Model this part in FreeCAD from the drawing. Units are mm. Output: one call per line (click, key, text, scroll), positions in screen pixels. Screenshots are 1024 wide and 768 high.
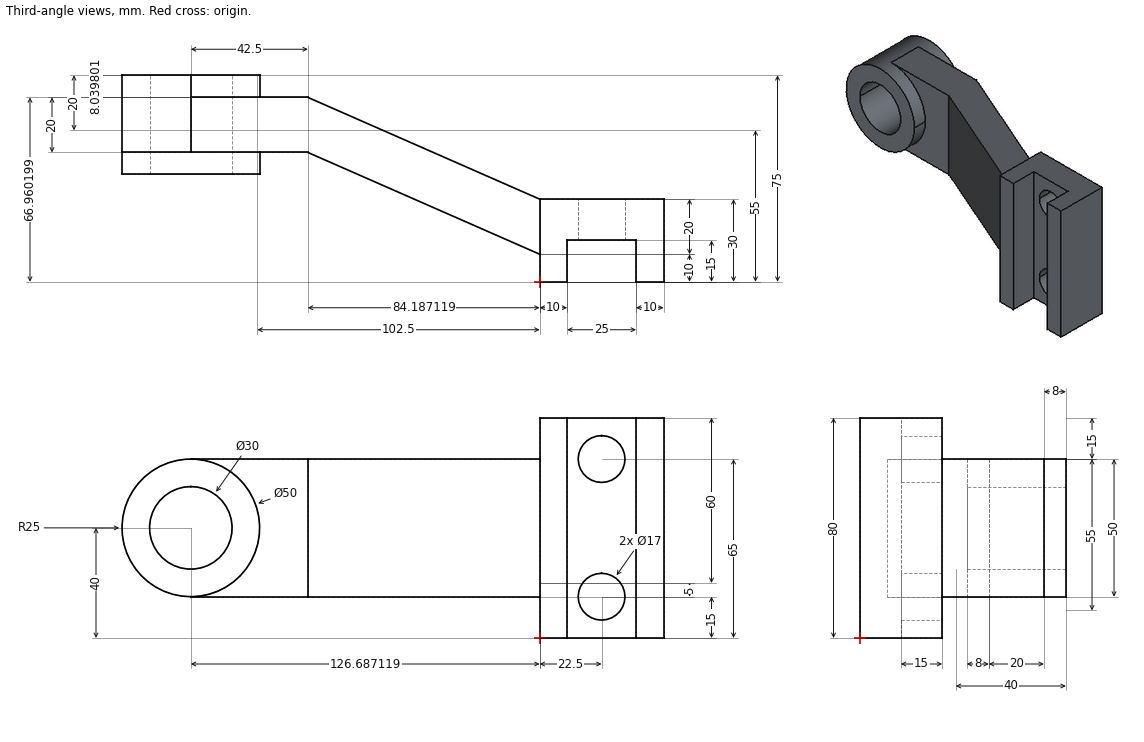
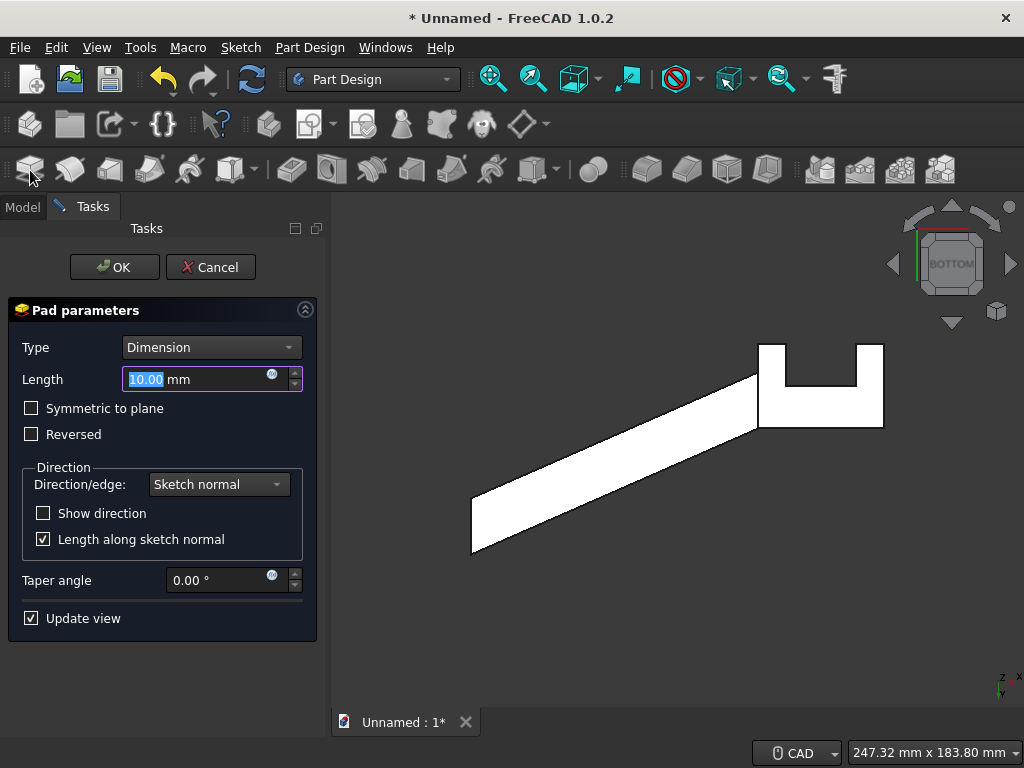
text(5)
key(Tab)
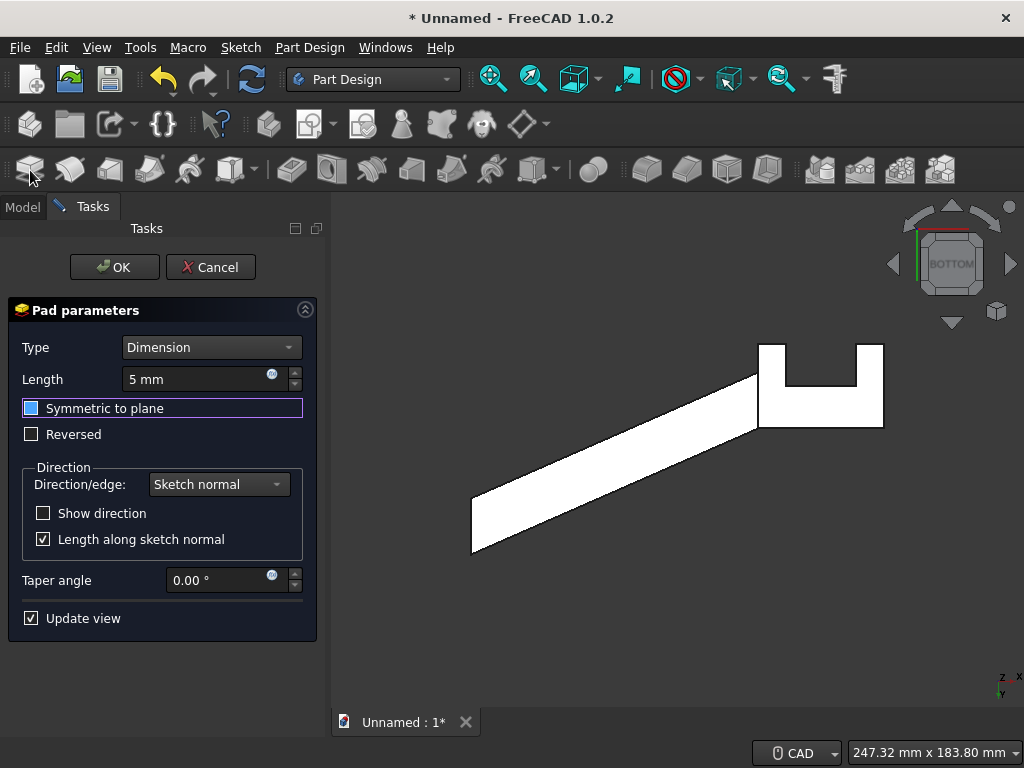
click(115, 267)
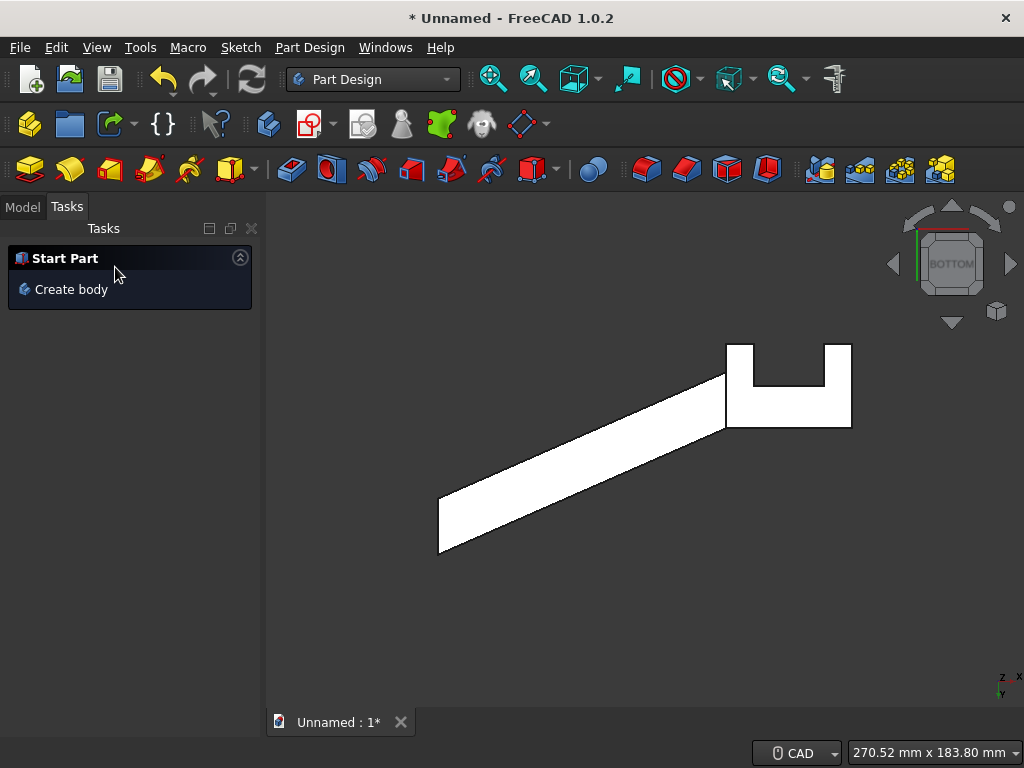
key(4)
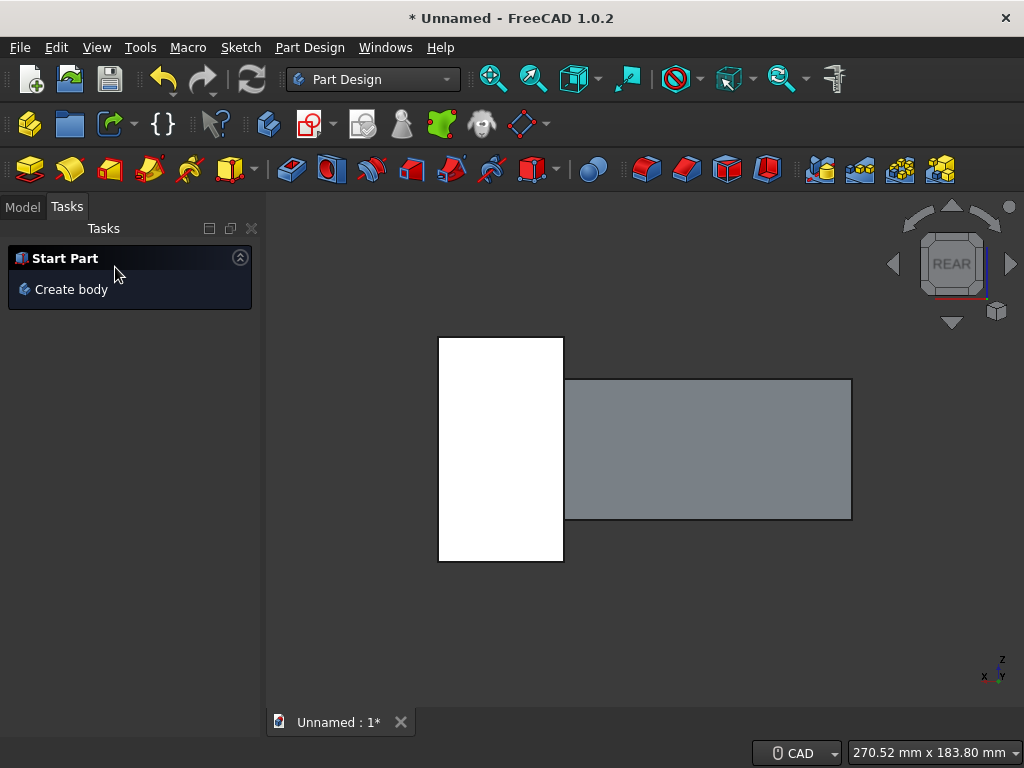
click(501, 416)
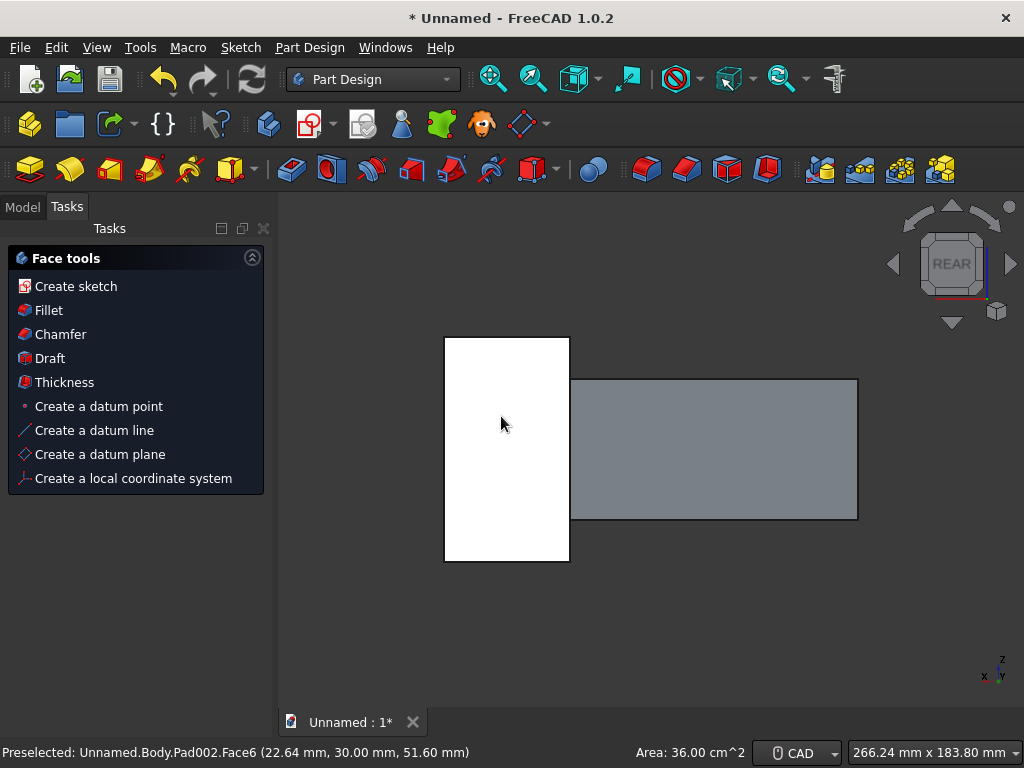
click(310, 124)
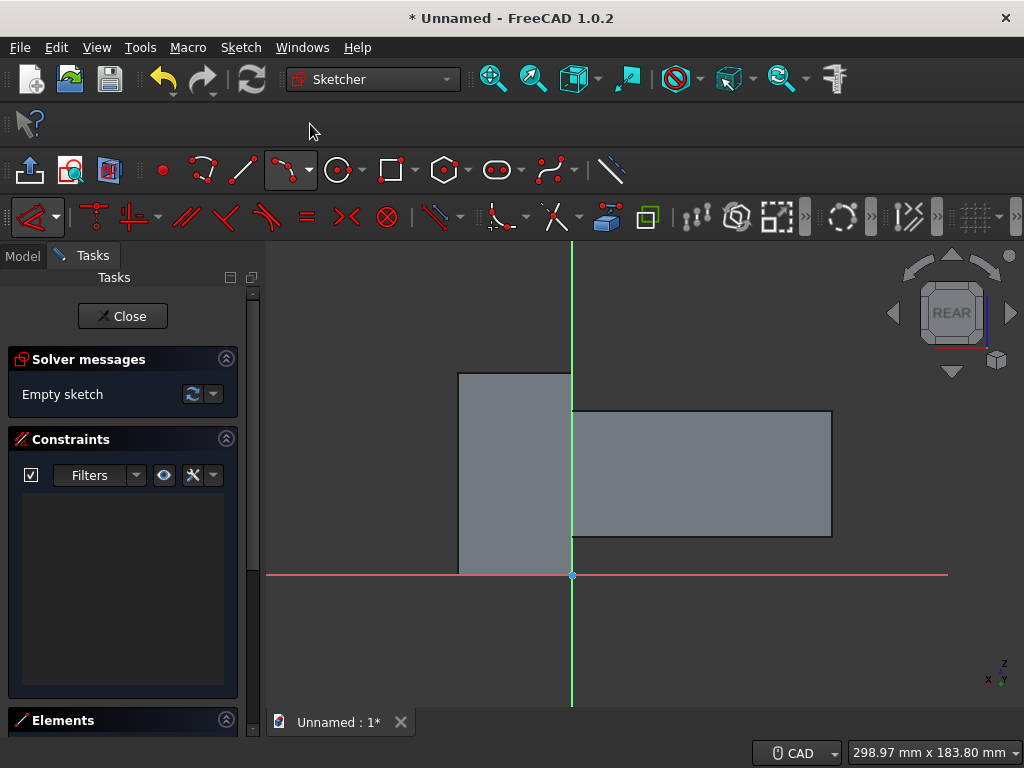
key(q)
key(s)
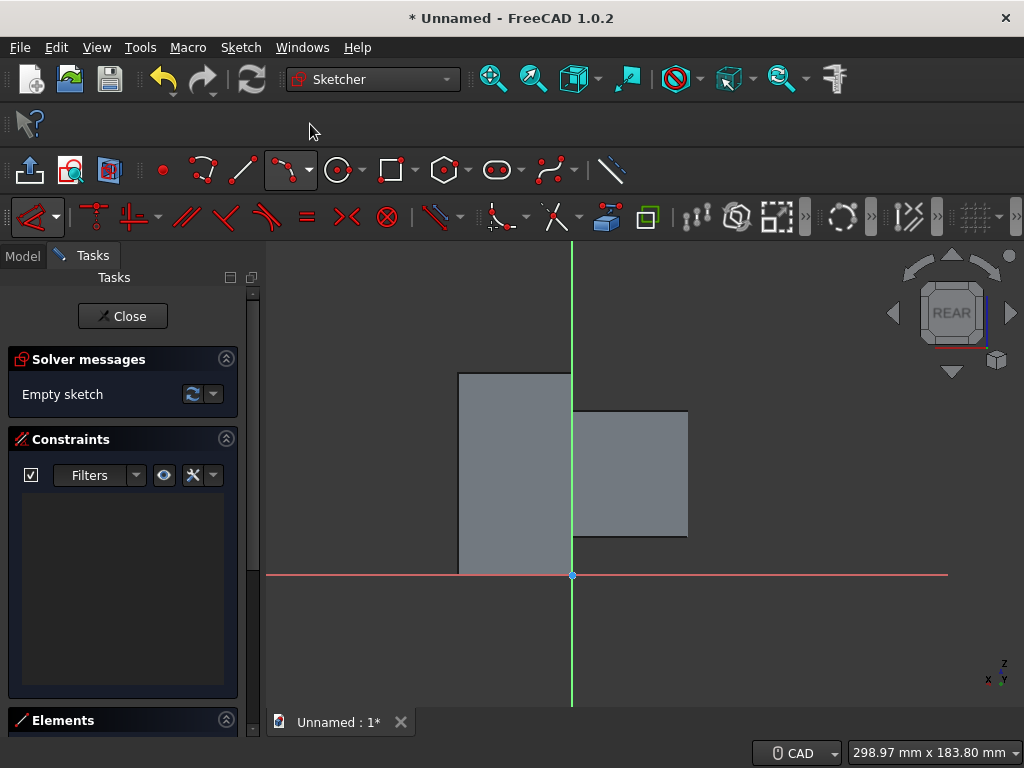
scroll(444, 499, up, 2)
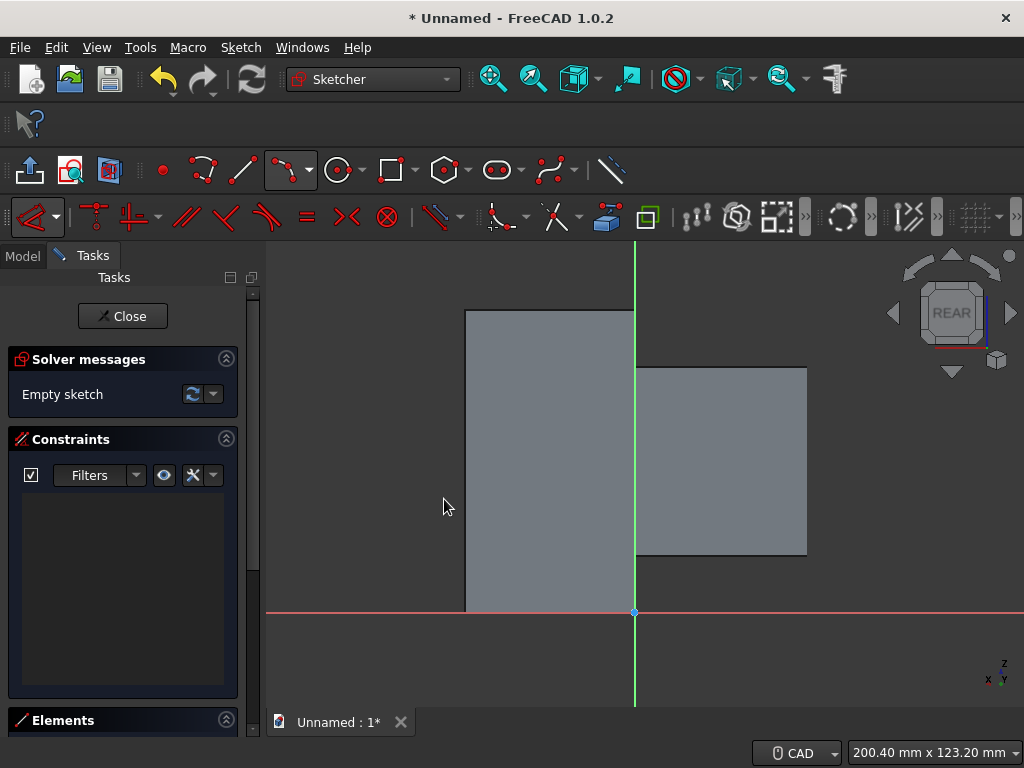
key(g)
key(c)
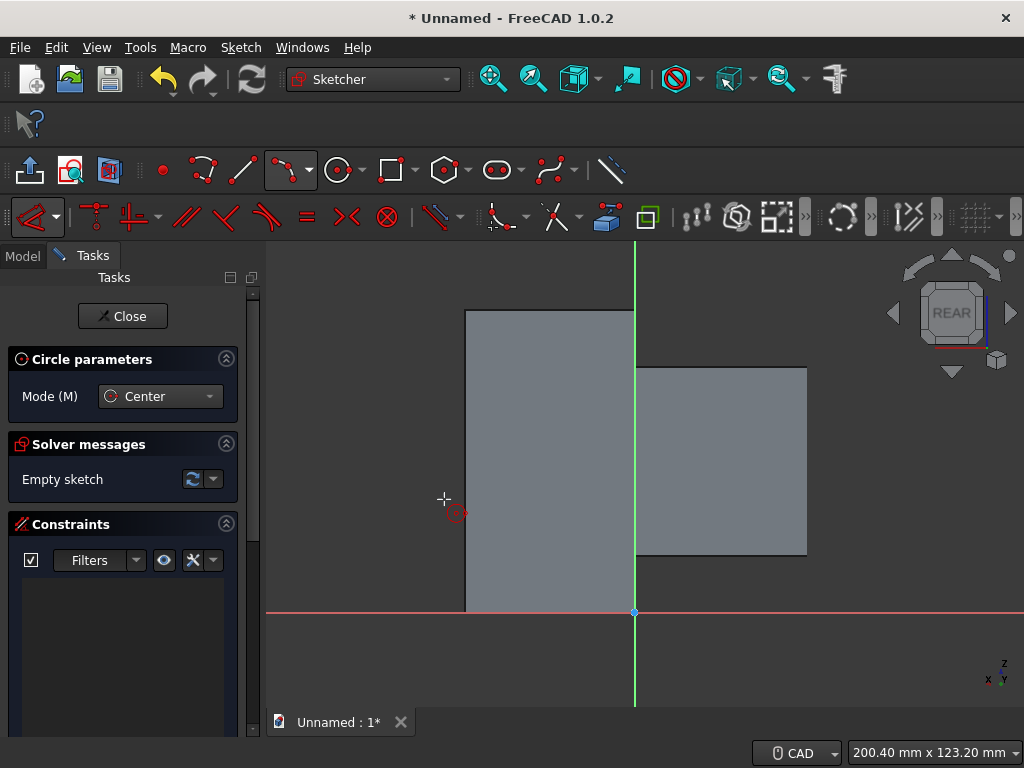
click(550, 556)
move(573, 533)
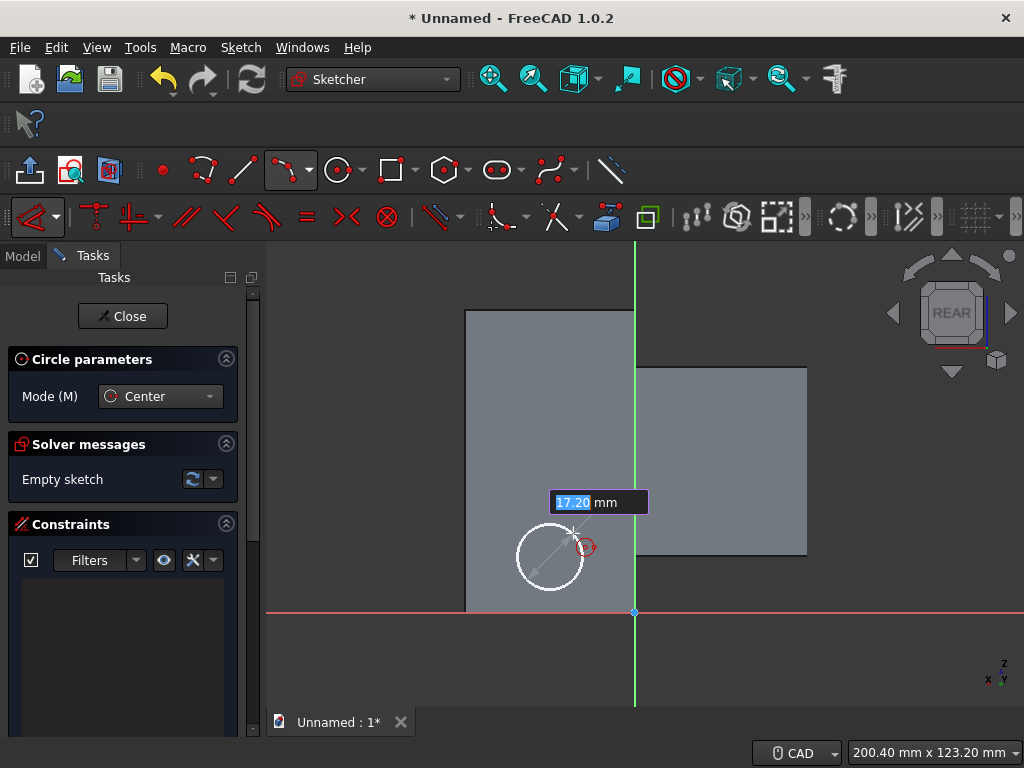
text(17)
key(Return)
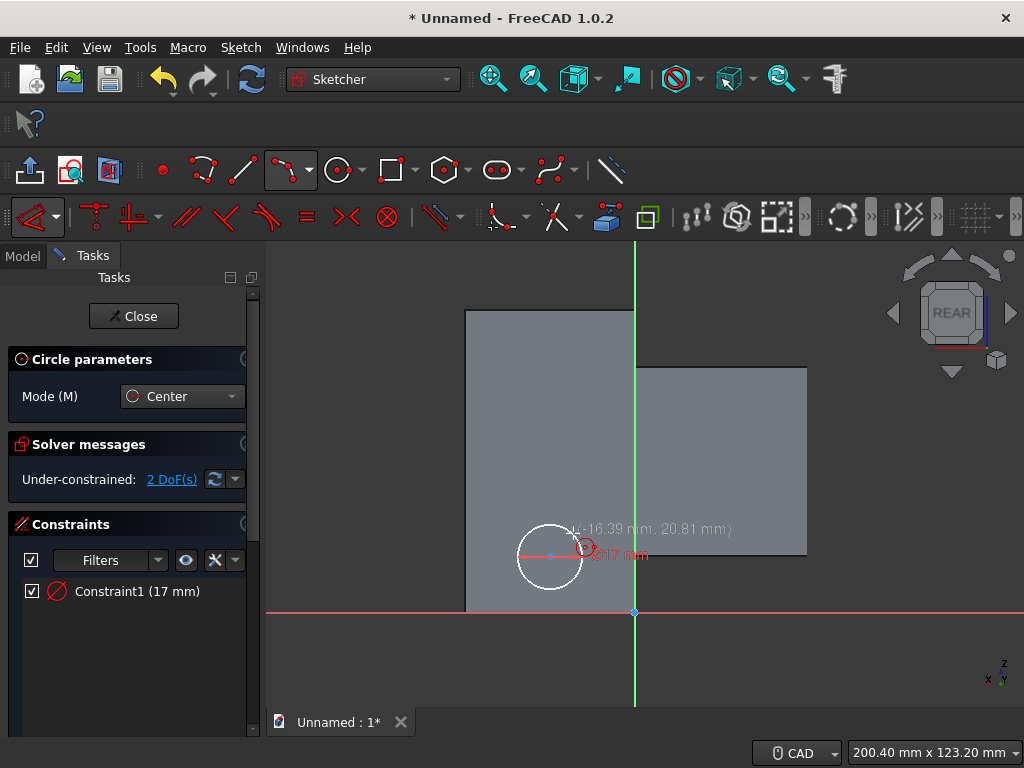
click(550, 367)
move(573, 344)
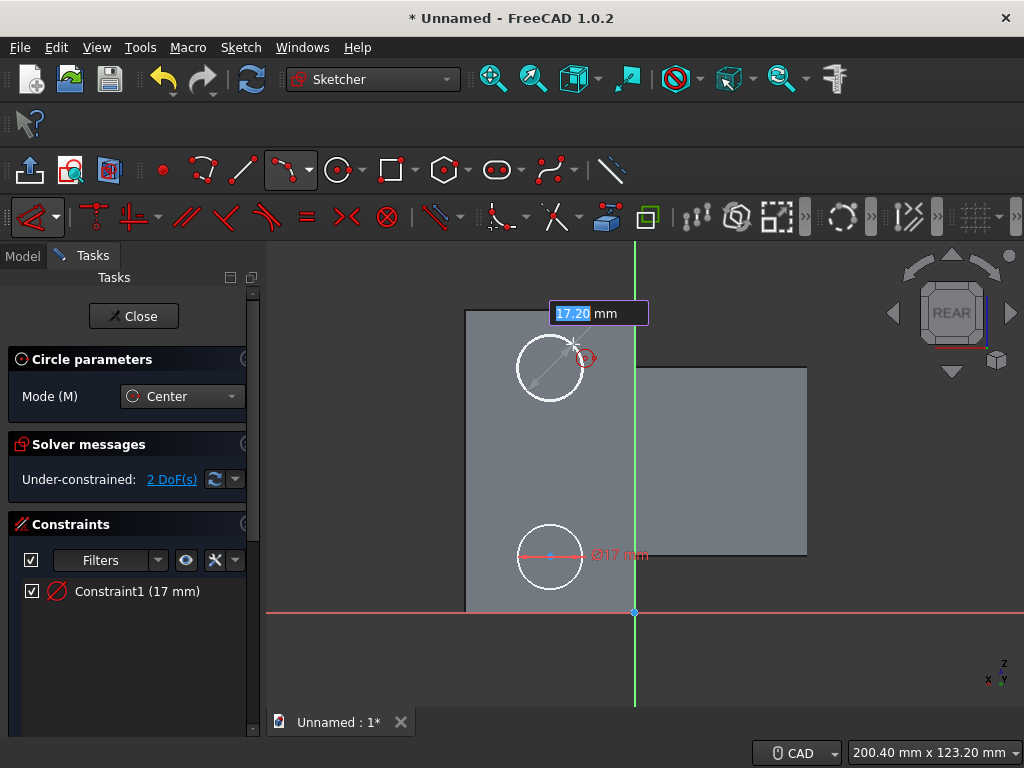
text(17)
key(Return)
key(Escape)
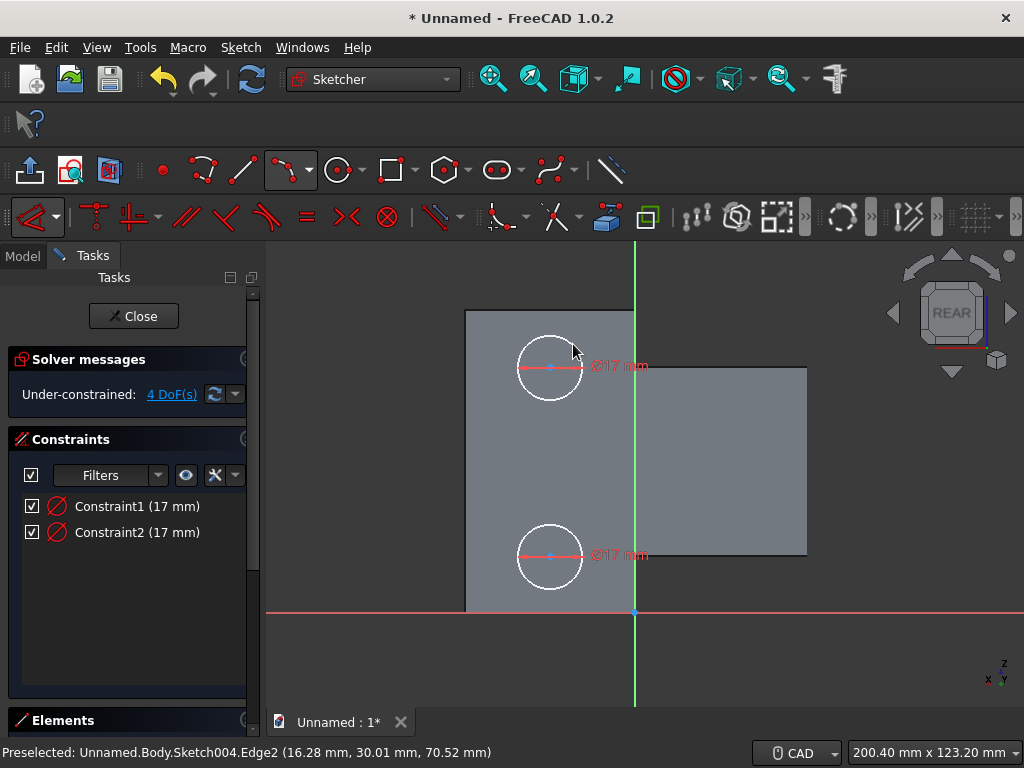
click(550, 557)